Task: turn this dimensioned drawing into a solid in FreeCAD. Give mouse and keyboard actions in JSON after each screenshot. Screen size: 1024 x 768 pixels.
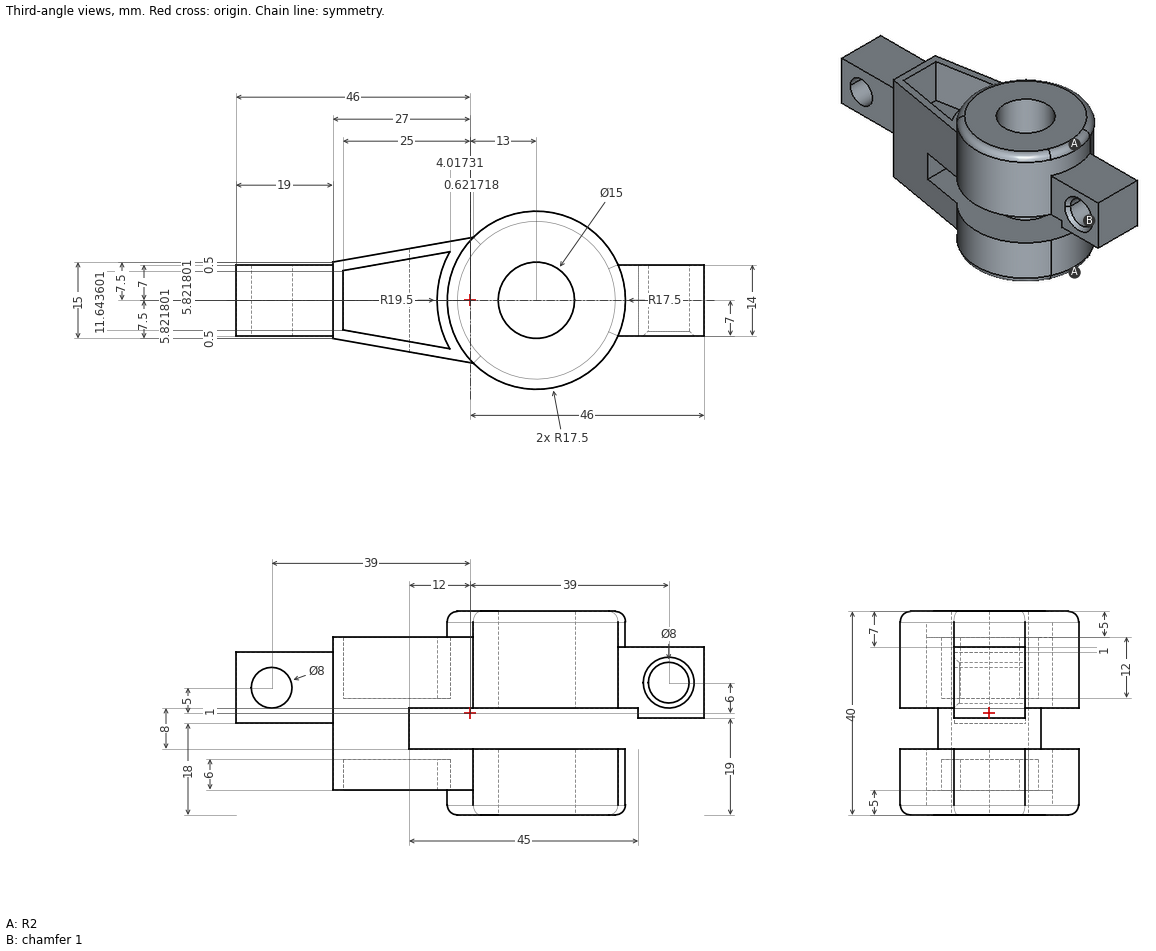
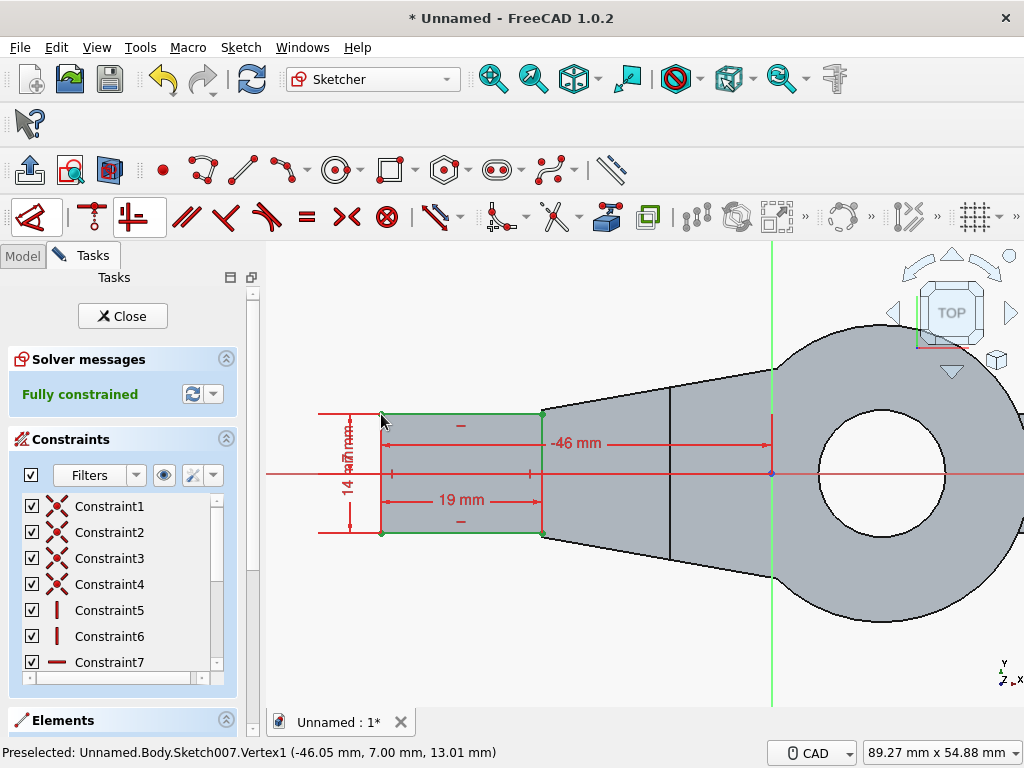
{"action": "left_click", "coordinate": [123, 316]}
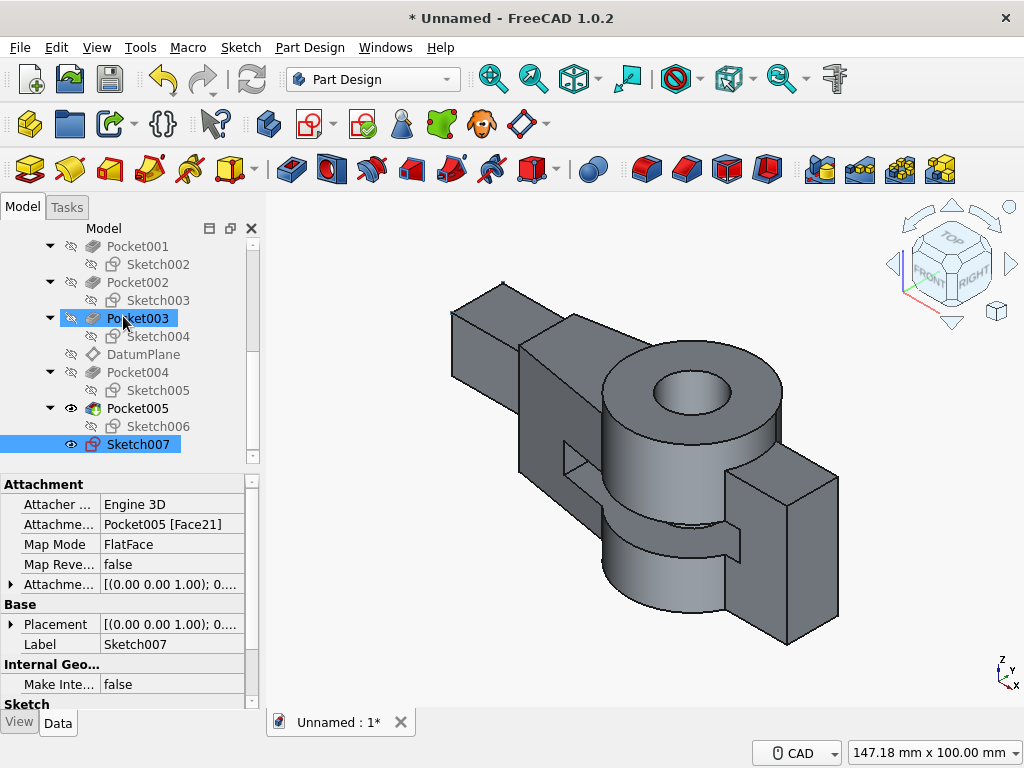
{"action": "left_click", "coordinate": [292, 170]}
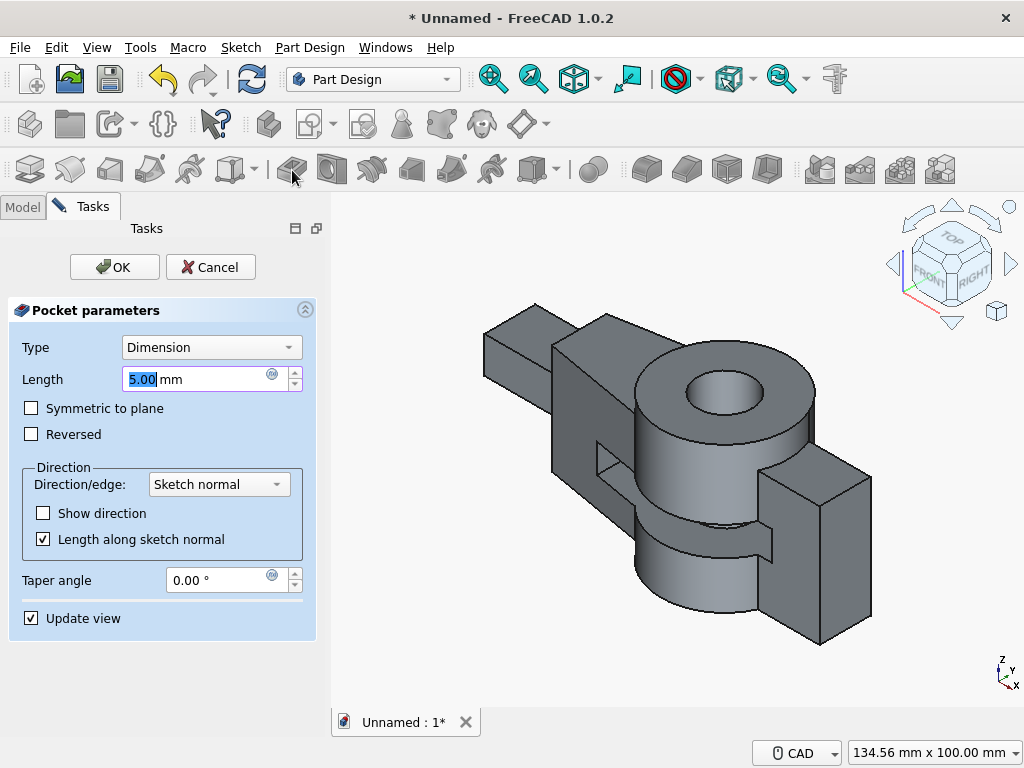
{"action": "type", "text": "1"}
{"action": "key", "text": "Tab"}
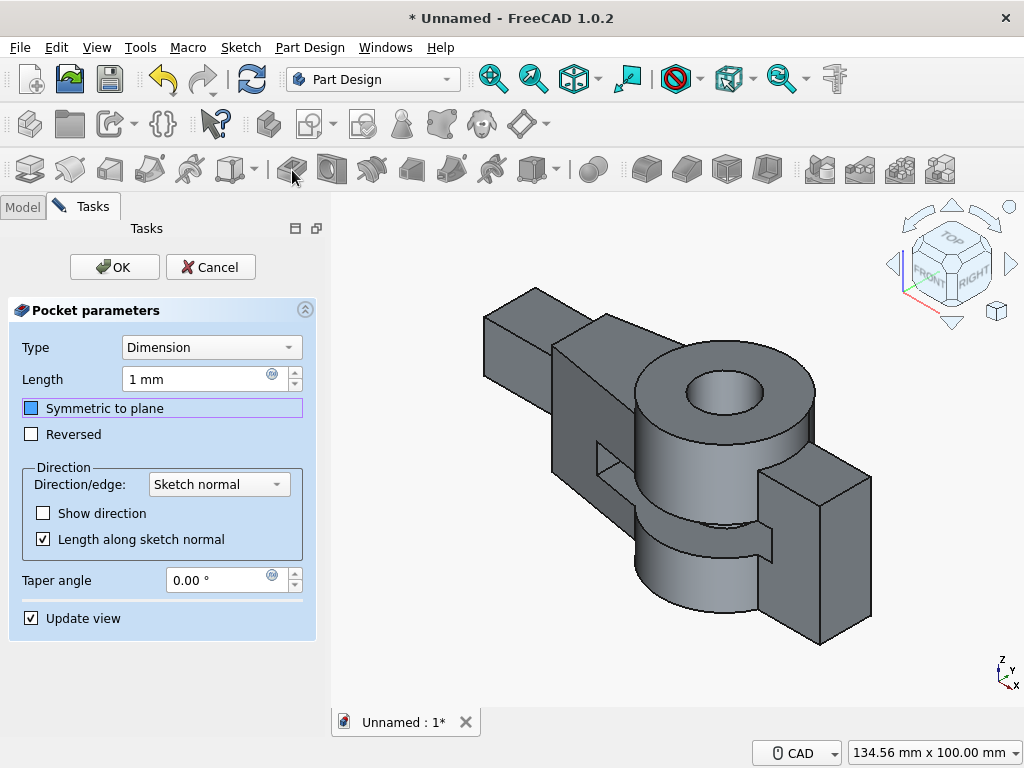
{"action": "left_click", "coordinate": [115, 267]}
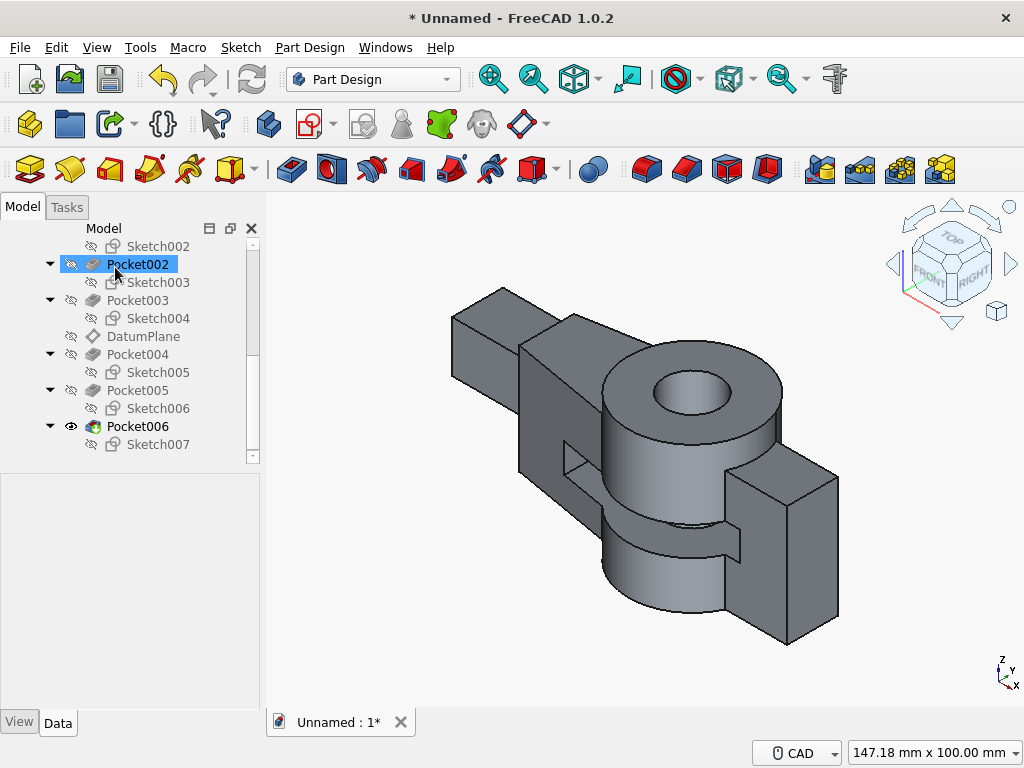
{"action": "scroll", "coordinate": [160, 350], "scroll_direction": "down", "scroll_amount": 3}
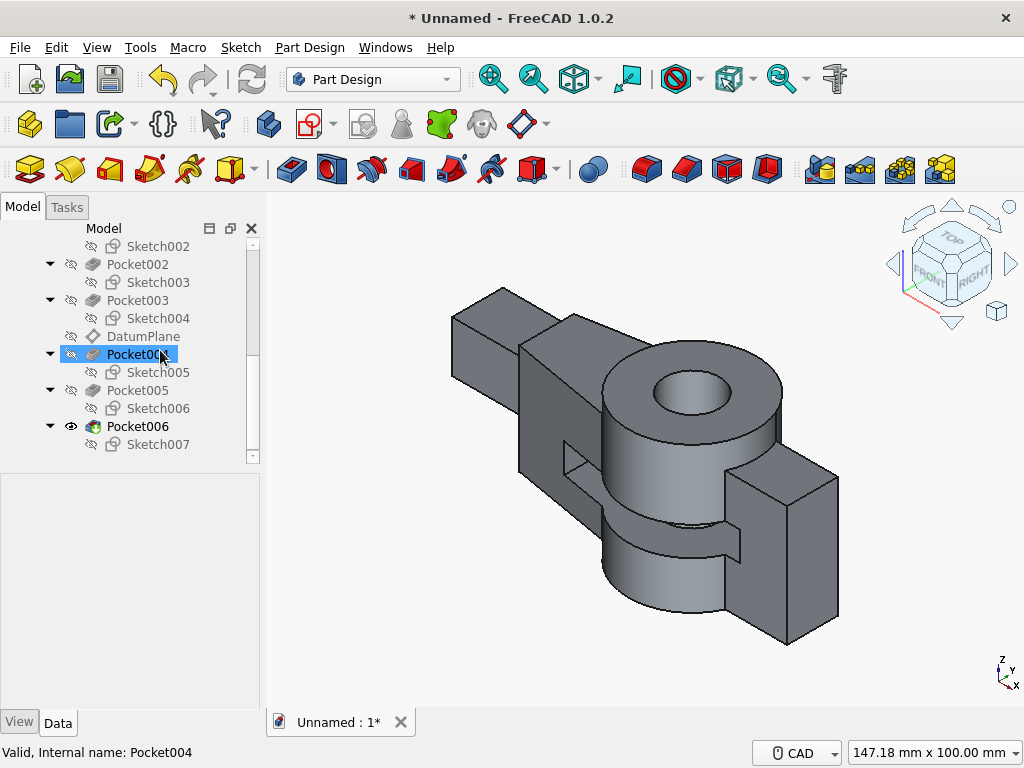
{"action": "scroll", "coordinate": [160, 350], "scroll_direction": "up", "scroll_amount": 15}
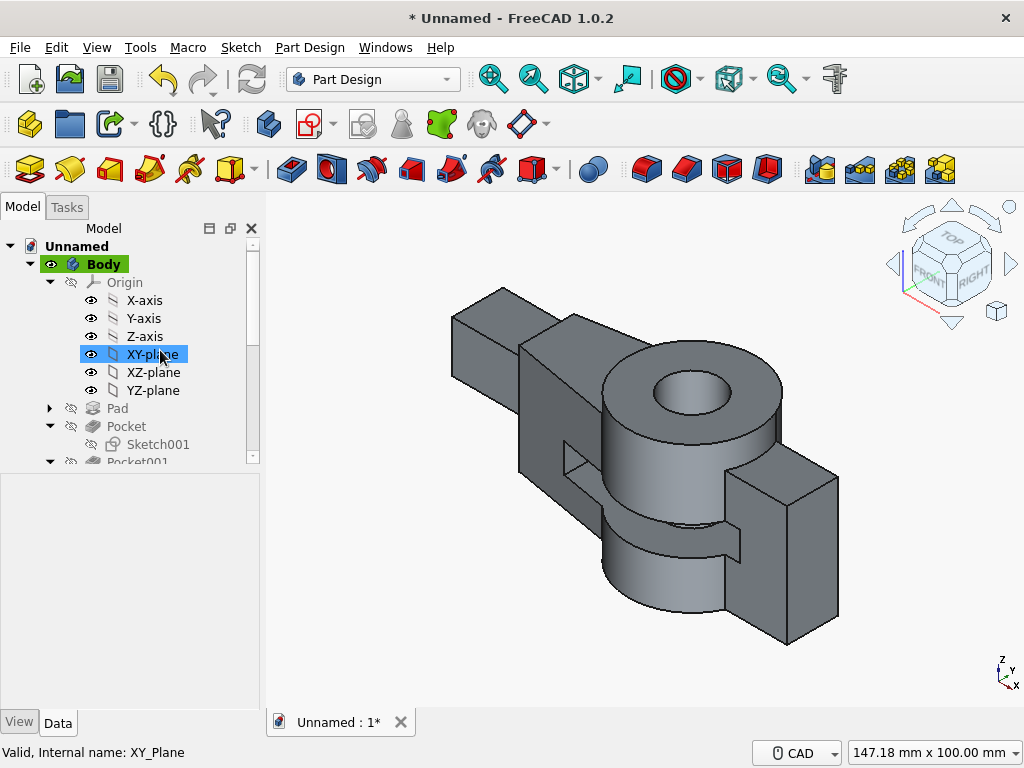
{"action": "left_click", "coordinate": [136, 354]}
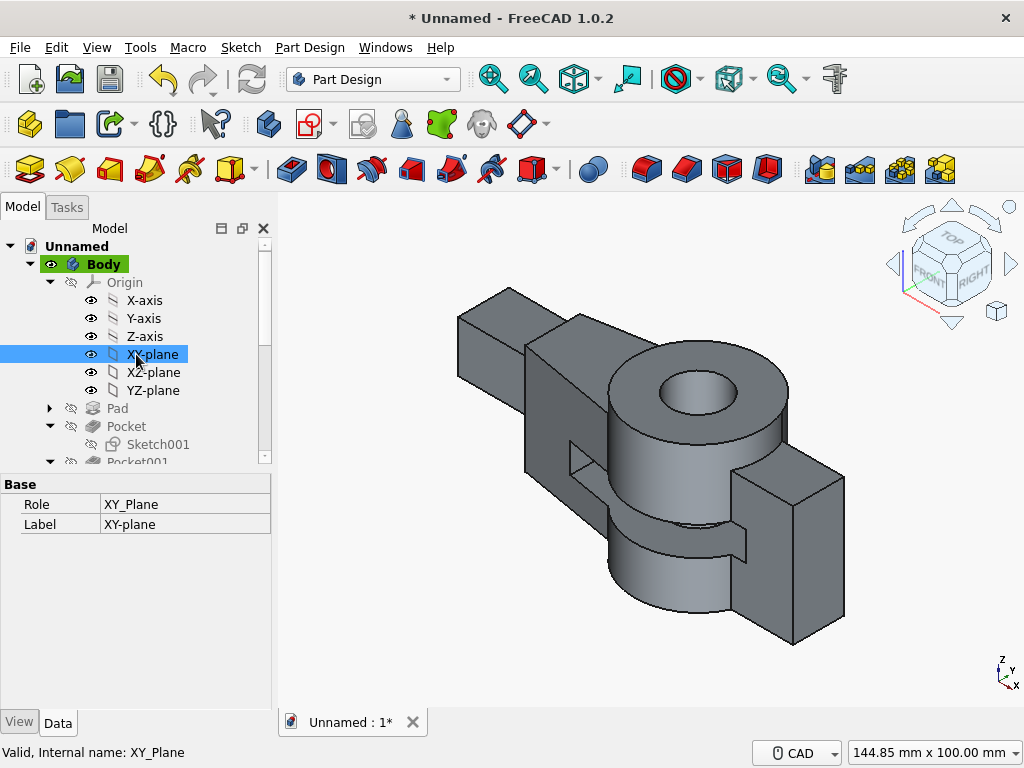
{"action": "left_click", "coordinate": [522, 124]}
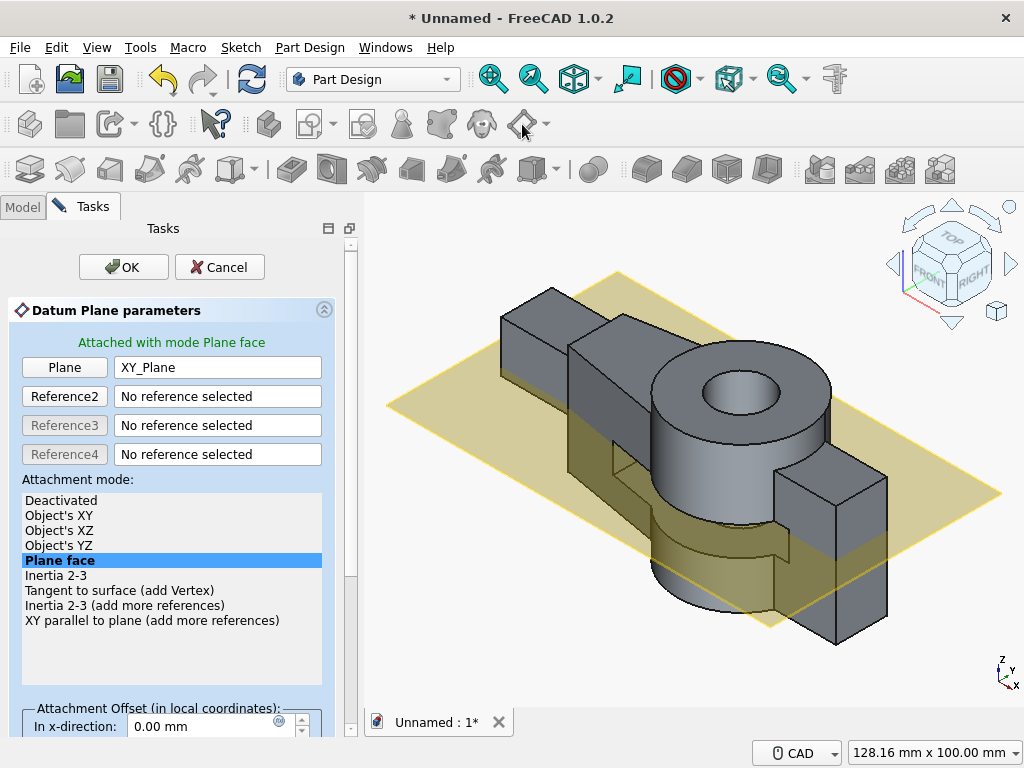
{"action": "scroll", "coordinate": [351, 487], "scroll_direction": "down", "scroll_amount": 3}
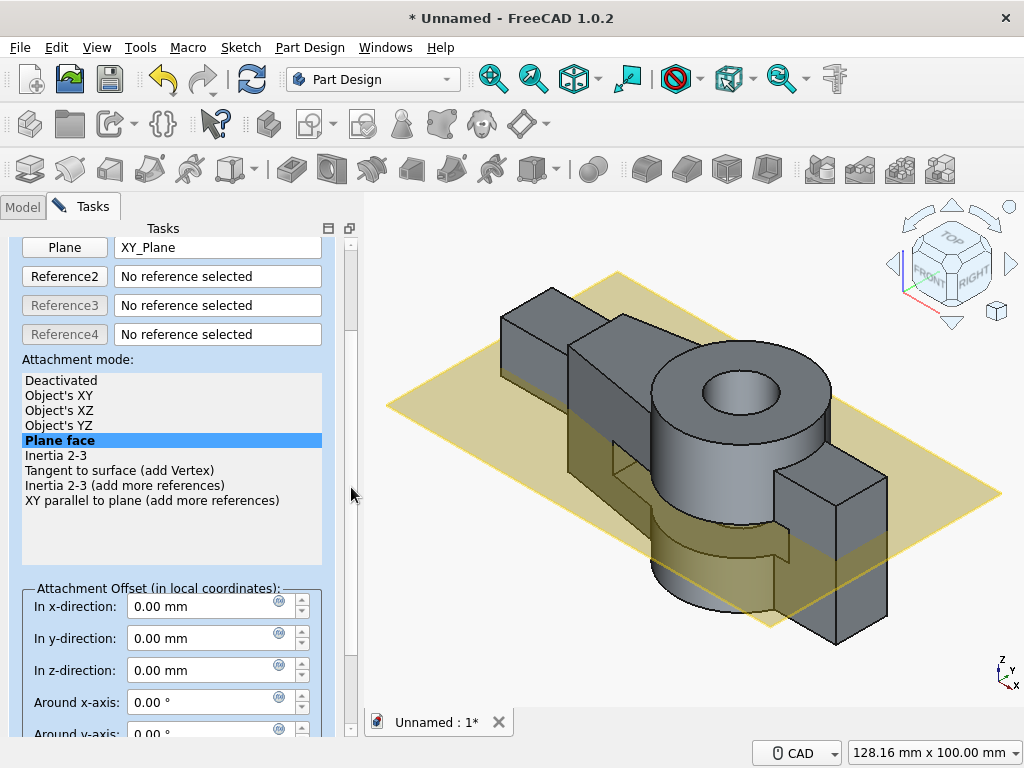
{"action": "triple_click", "coordinate": [210, 610]}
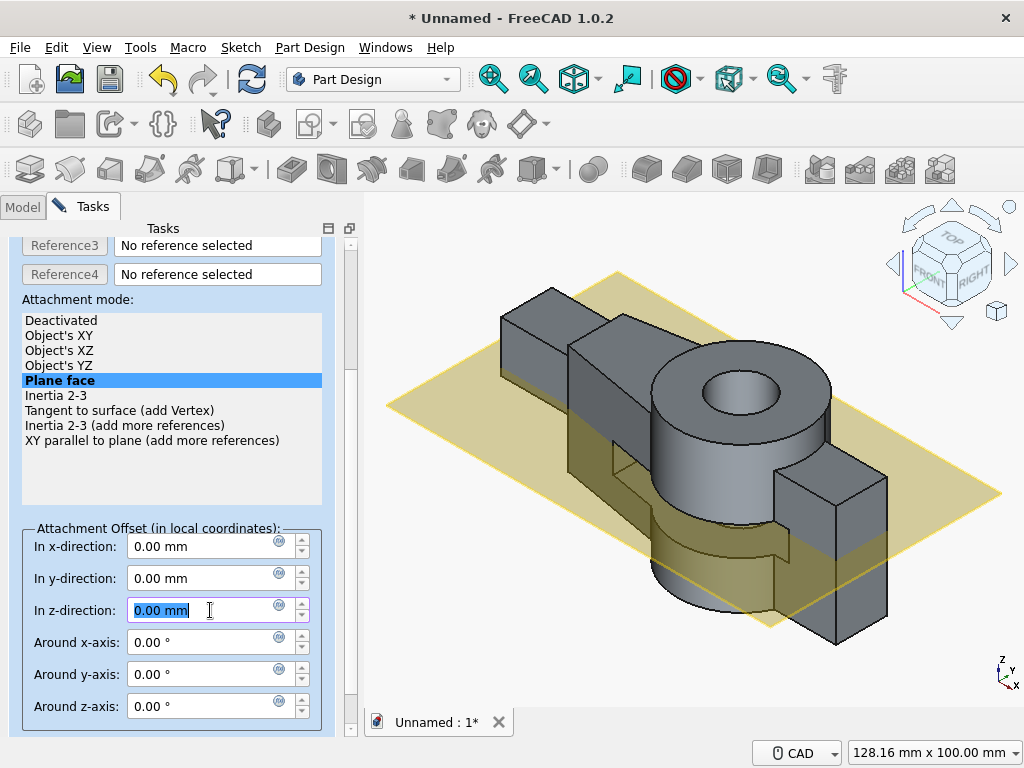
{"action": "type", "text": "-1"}
{"action": "key", "text": "Tab"}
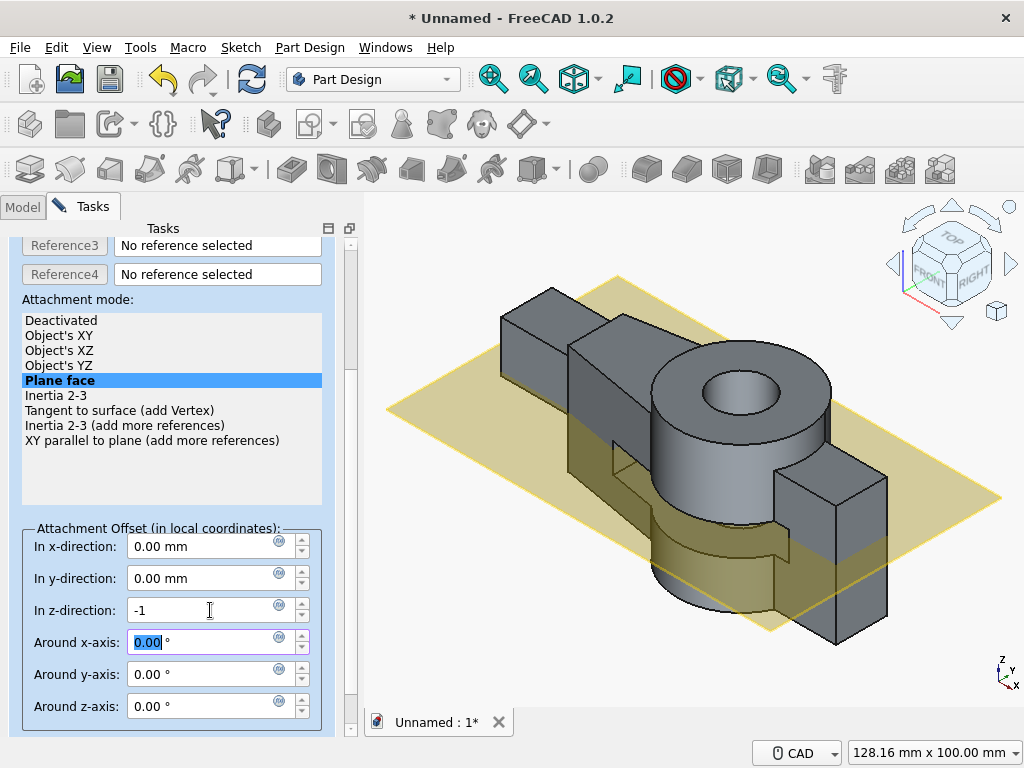
{"action": "scroll", "coordinate": [351, 487], "scroll_direction": "up", "scroll_amount": 4}